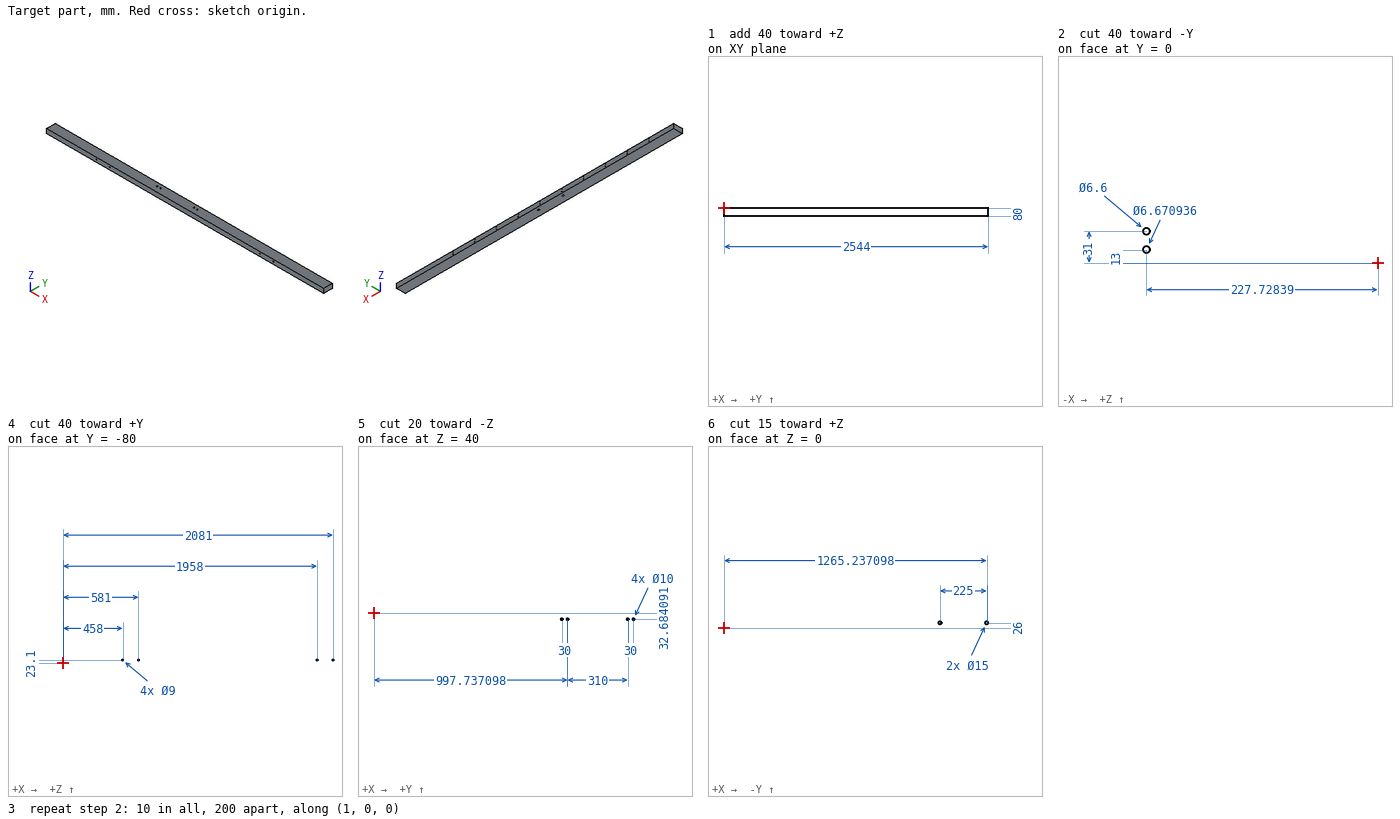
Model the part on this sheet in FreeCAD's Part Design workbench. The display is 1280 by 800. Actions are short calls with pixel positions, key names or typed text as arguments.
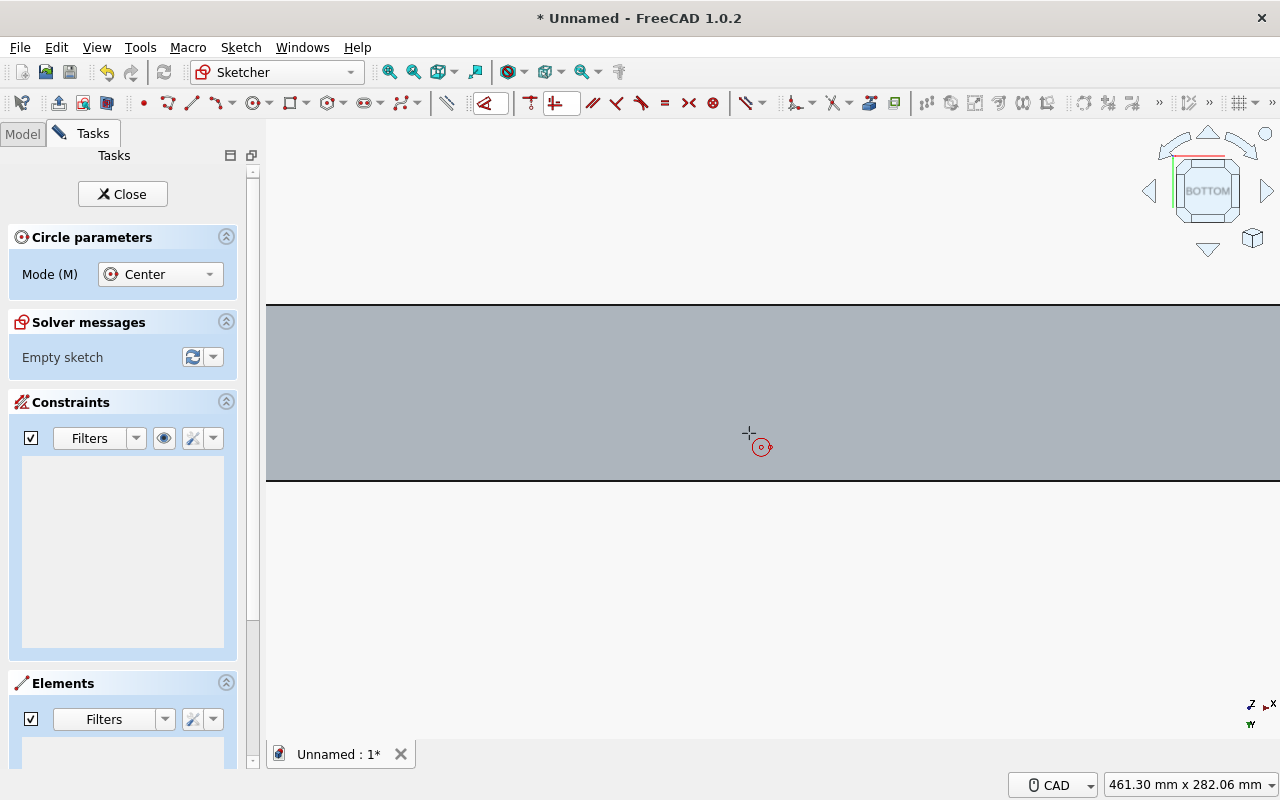
scroll(947, 424, up, 2)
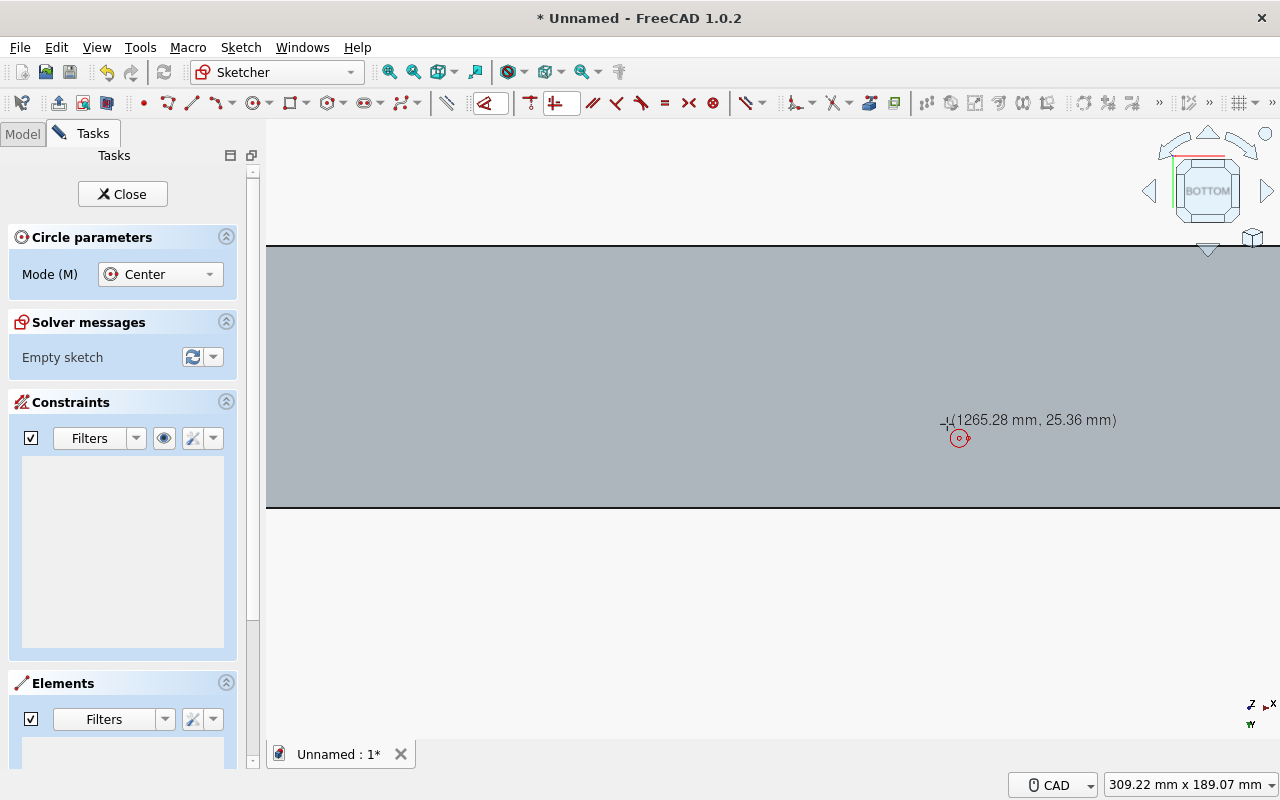
click(947, 423)
move(964, 406)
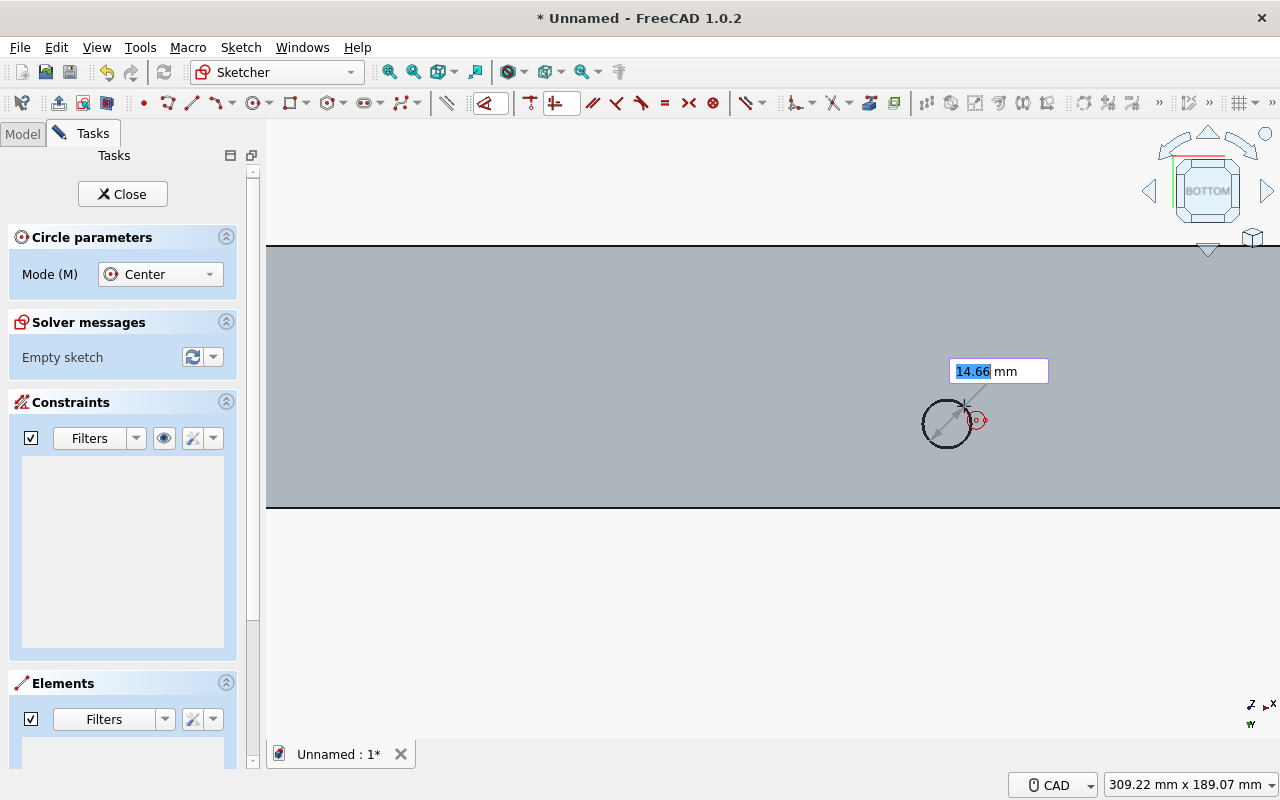
text(15)
key(Return)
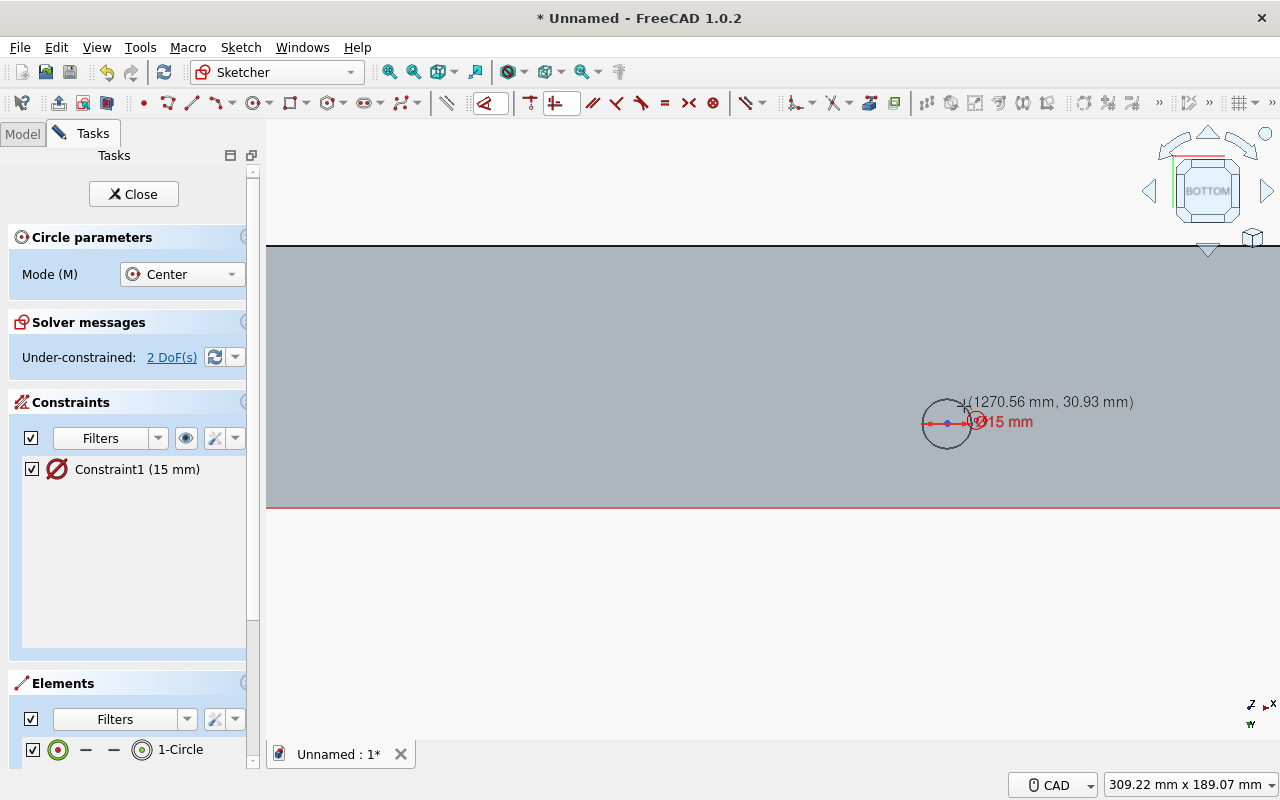
scroll(962, 441, down, 2)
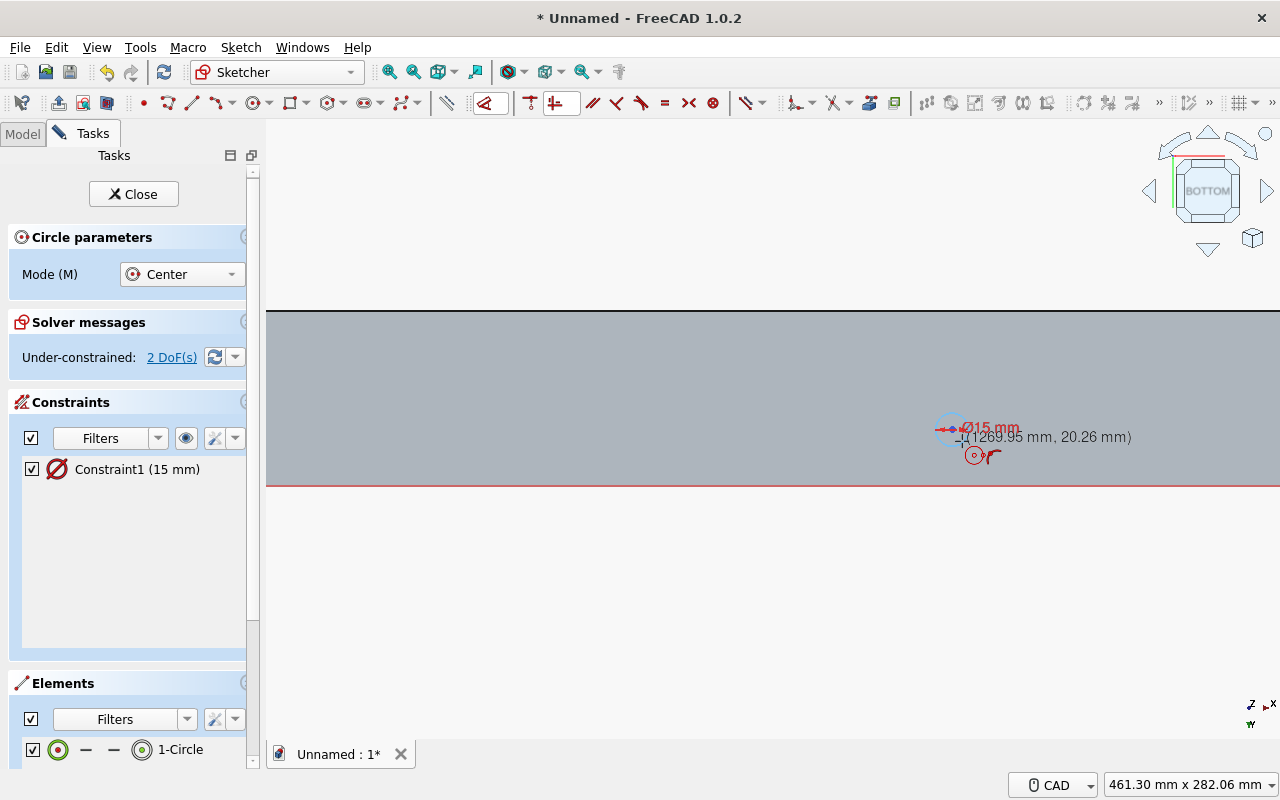
scroll(457, 429, up, 2)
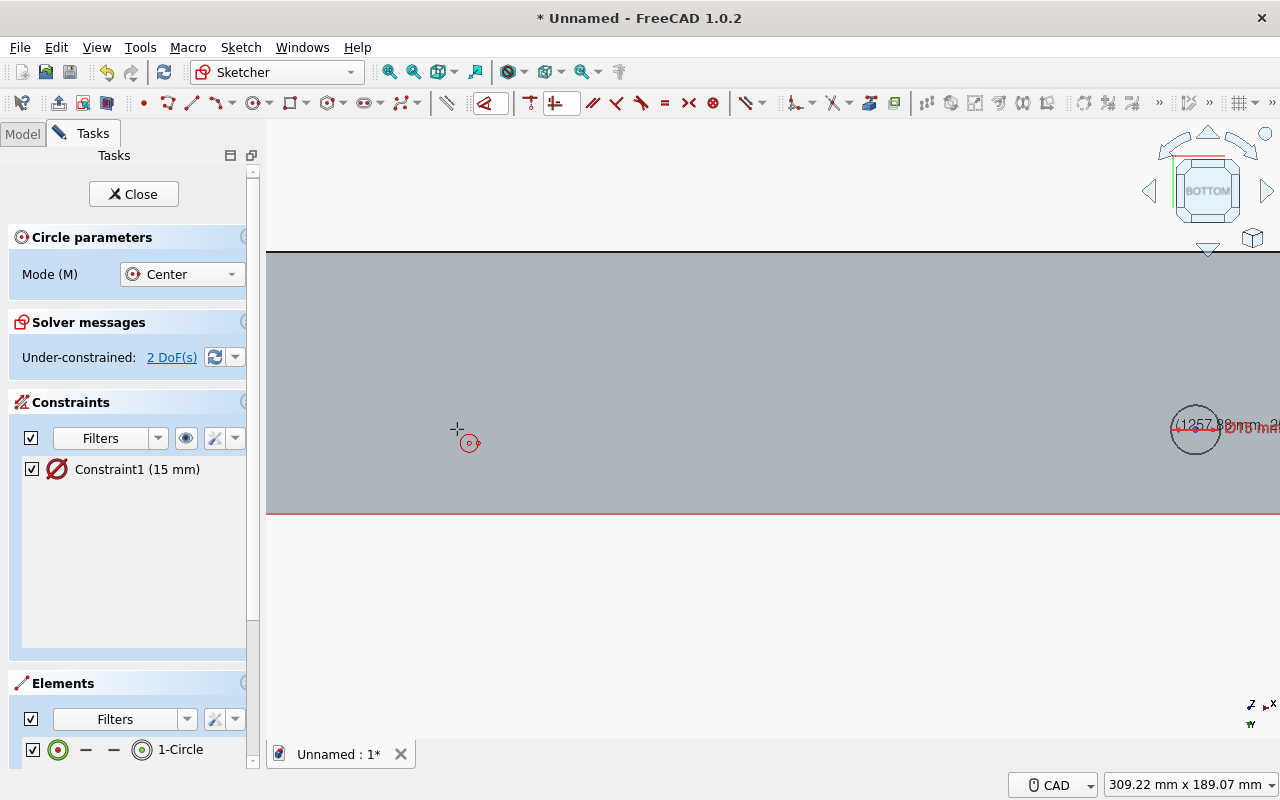
click(457, 429)
move(475, 412)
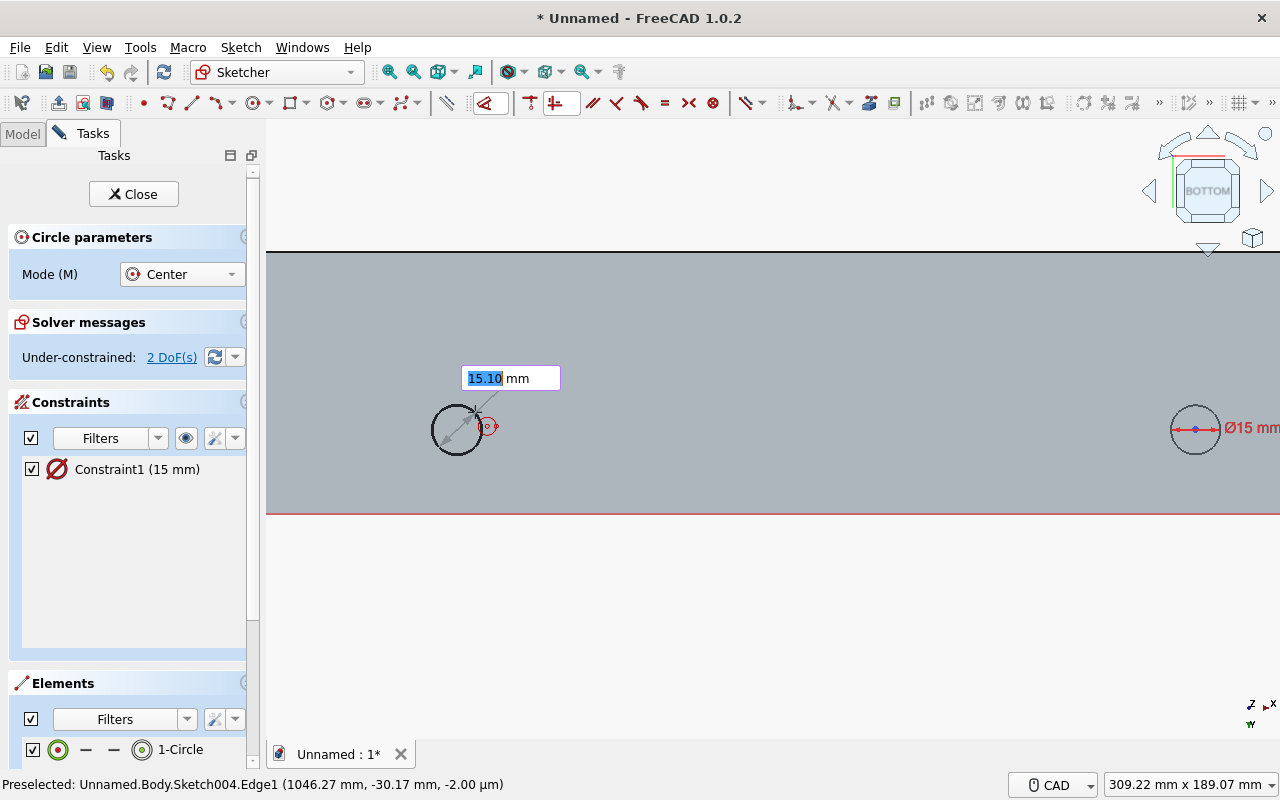
text(15)
key(Return)
key(Escape)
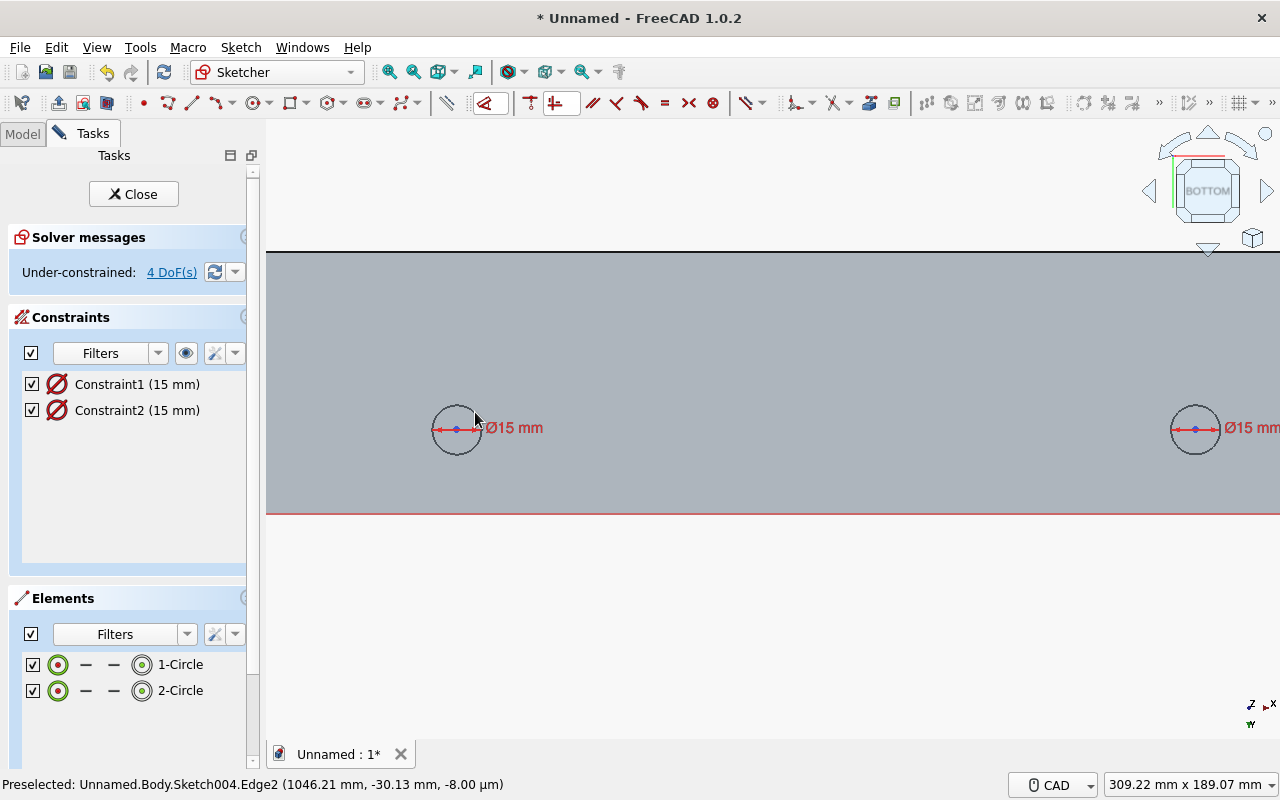
scroll(457, 429, down, 2)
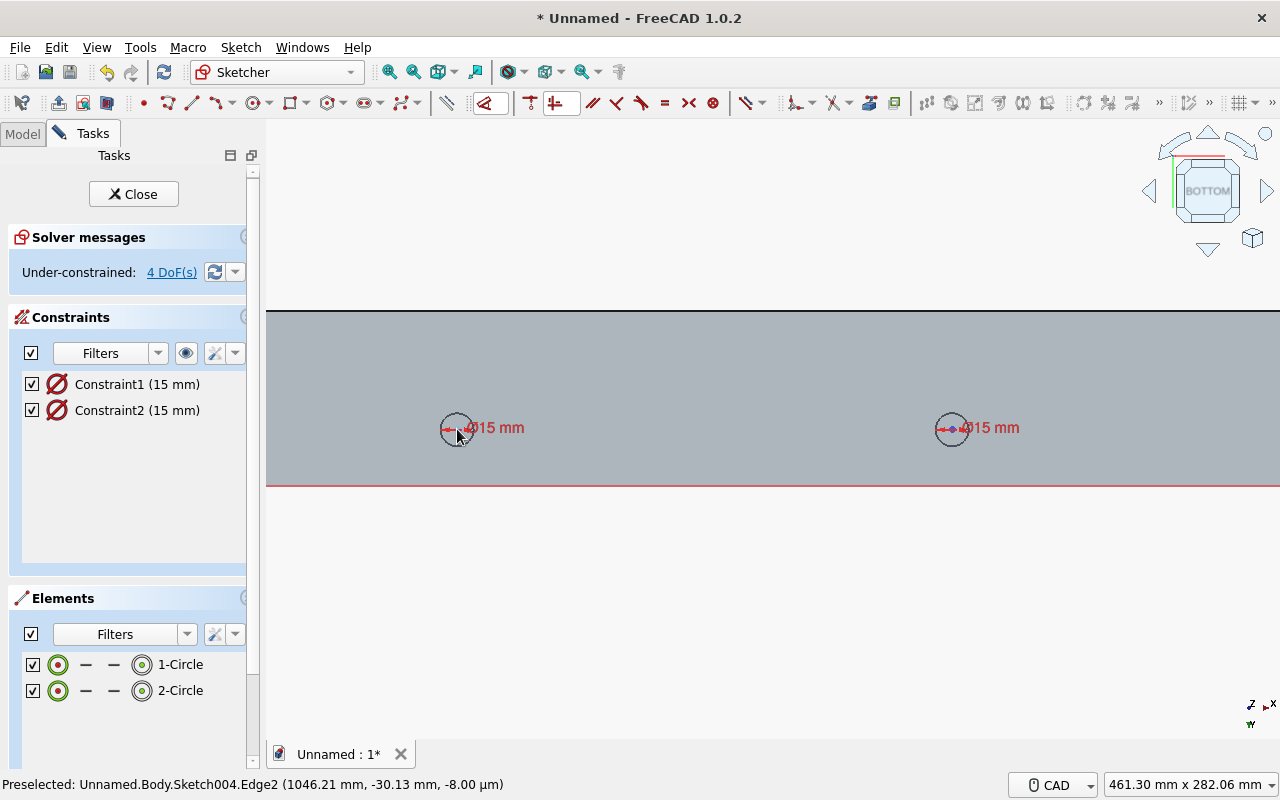
click(952, 430)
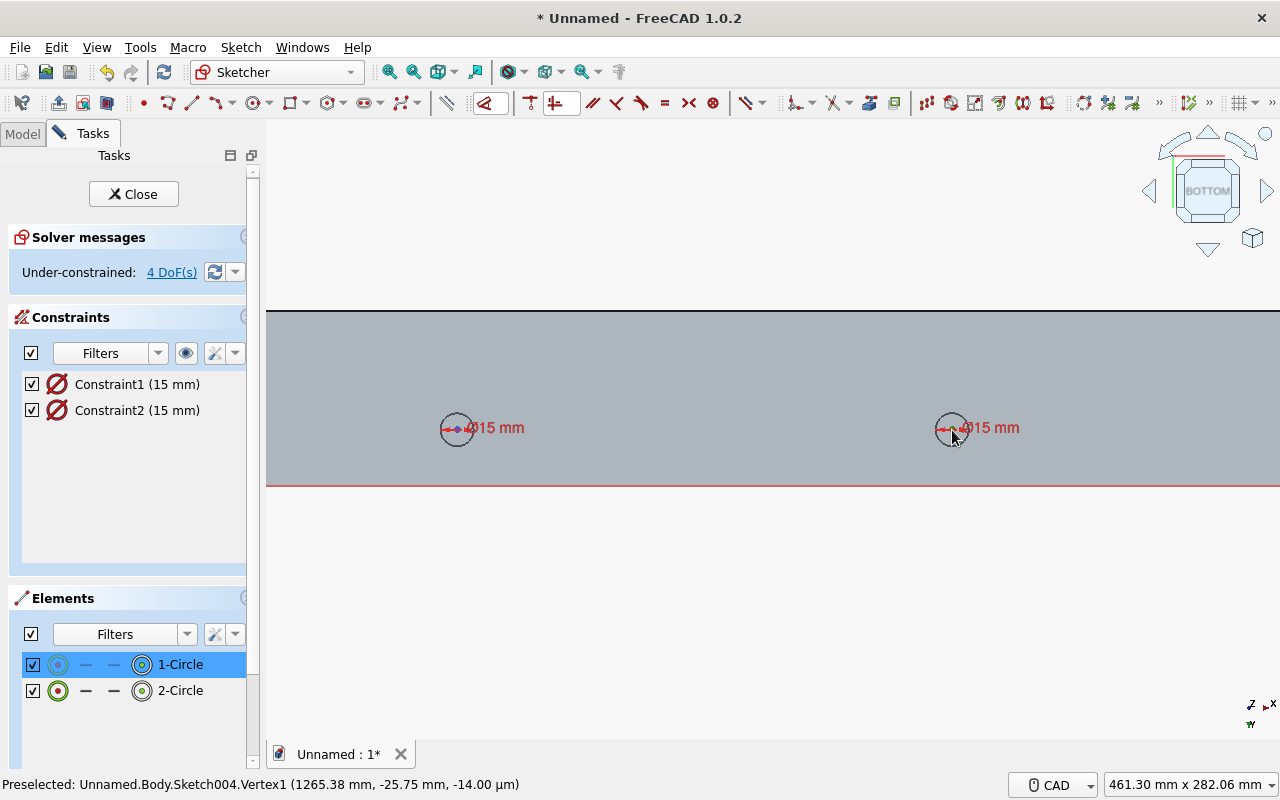
click(457, 430)